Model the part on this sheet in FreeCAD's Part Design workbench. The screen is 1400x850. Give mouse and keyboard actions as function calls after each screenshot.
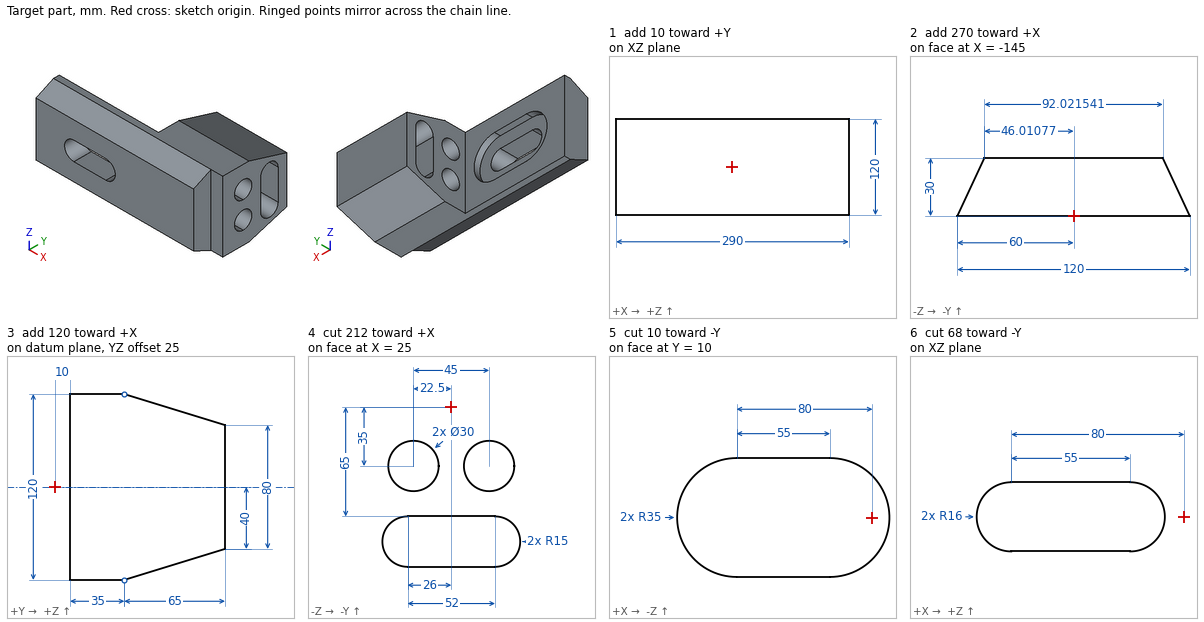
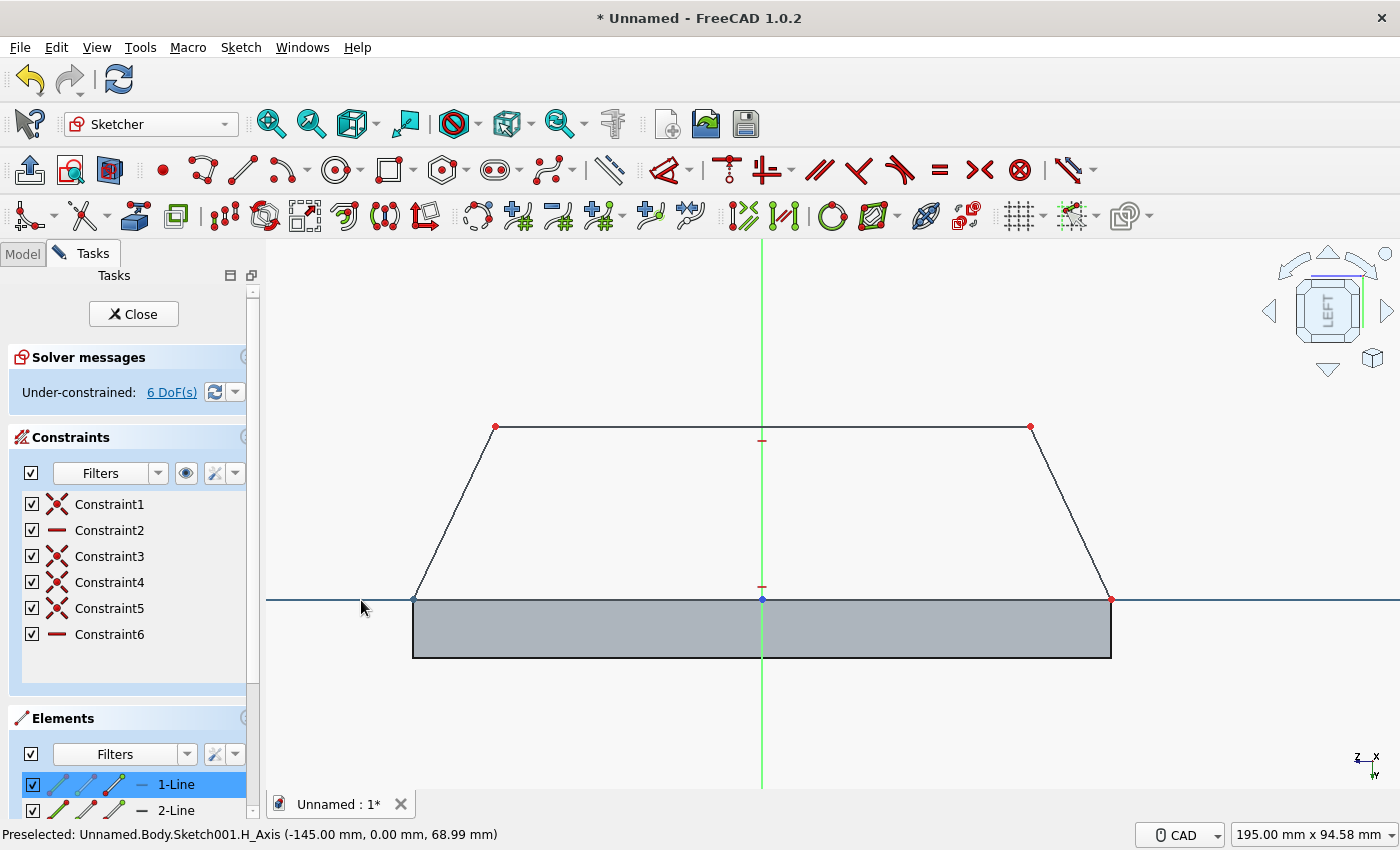
key(c)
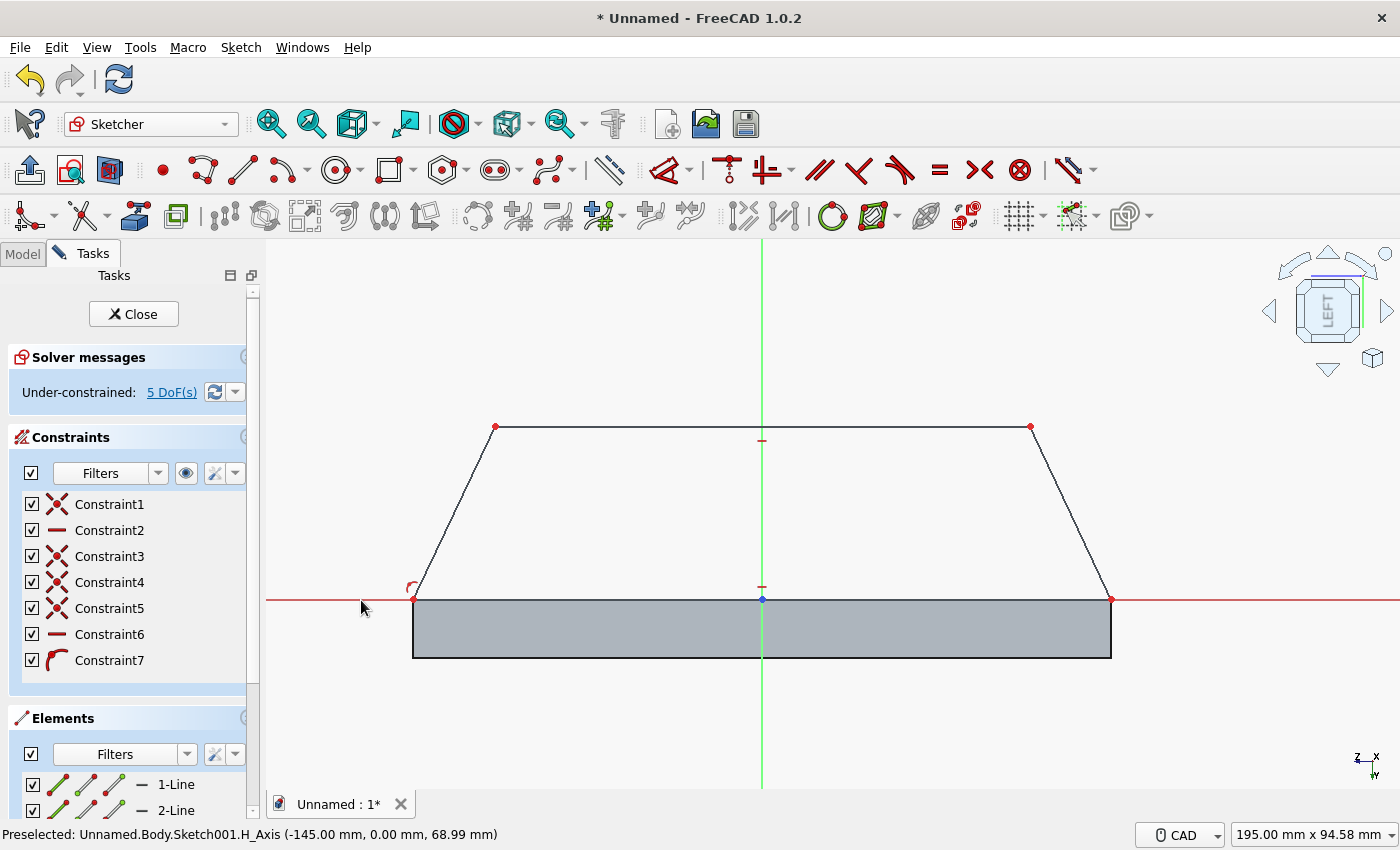
key(d)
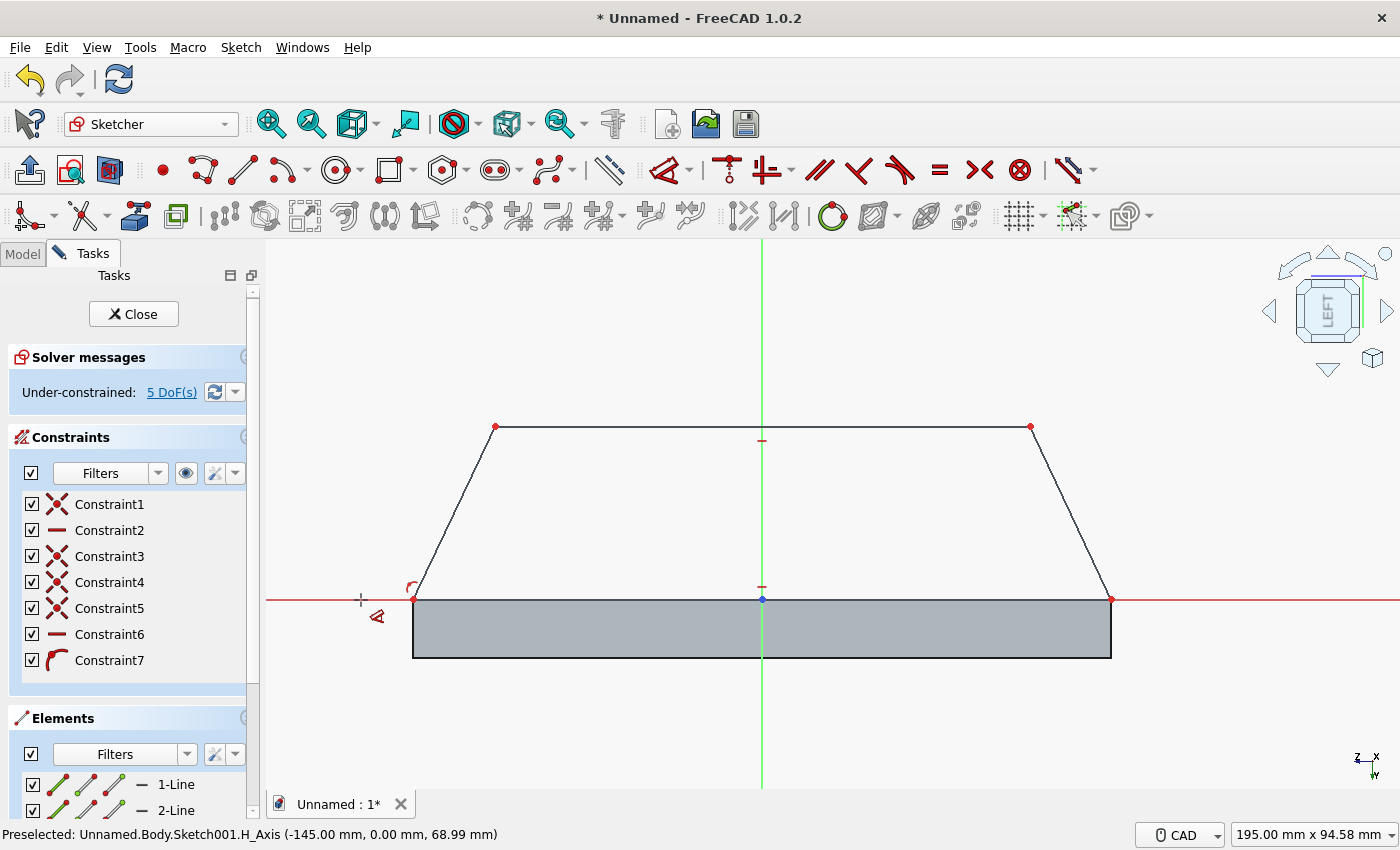
click(622, 600)
click(601, 634)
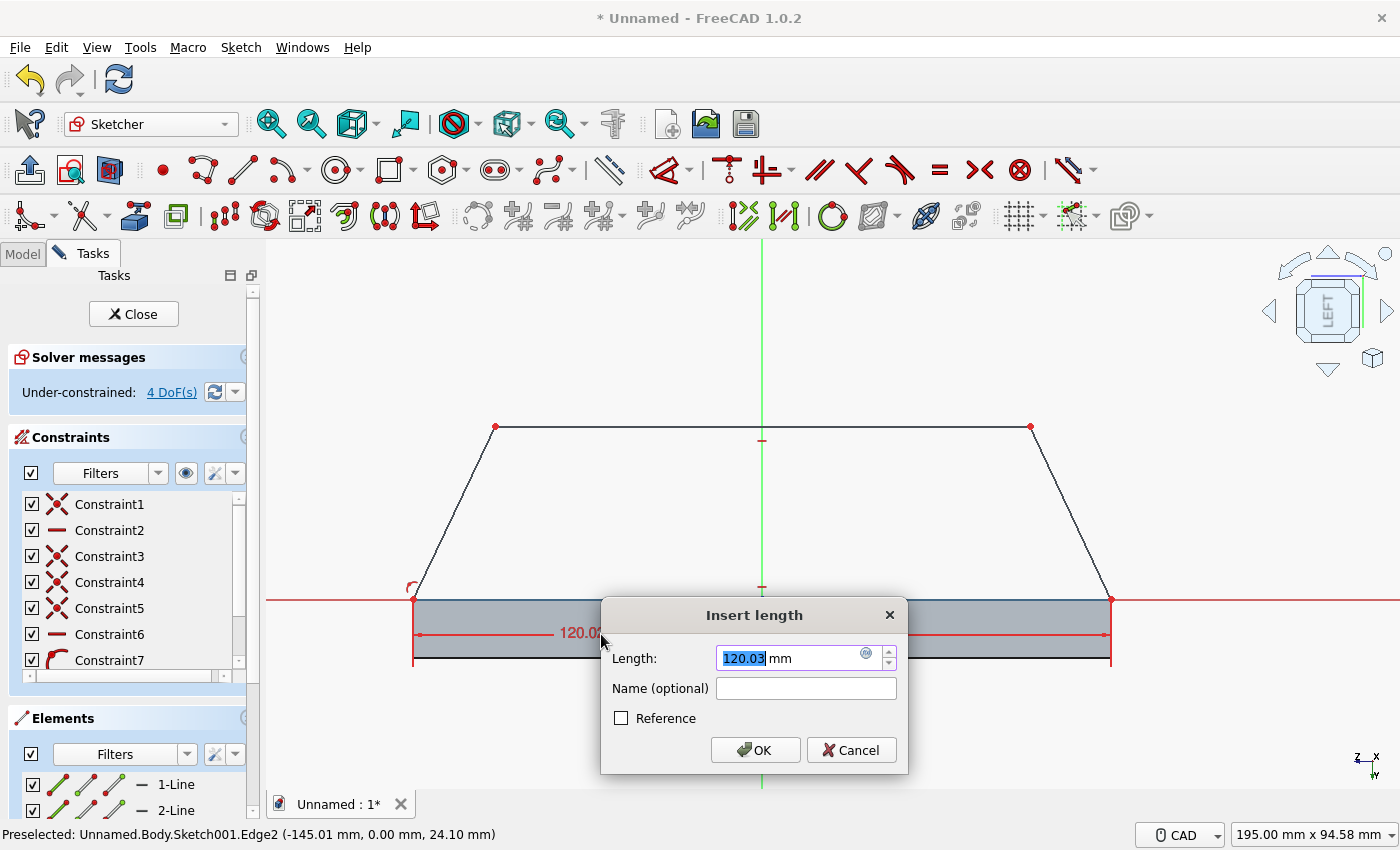
text(120)
key(Return)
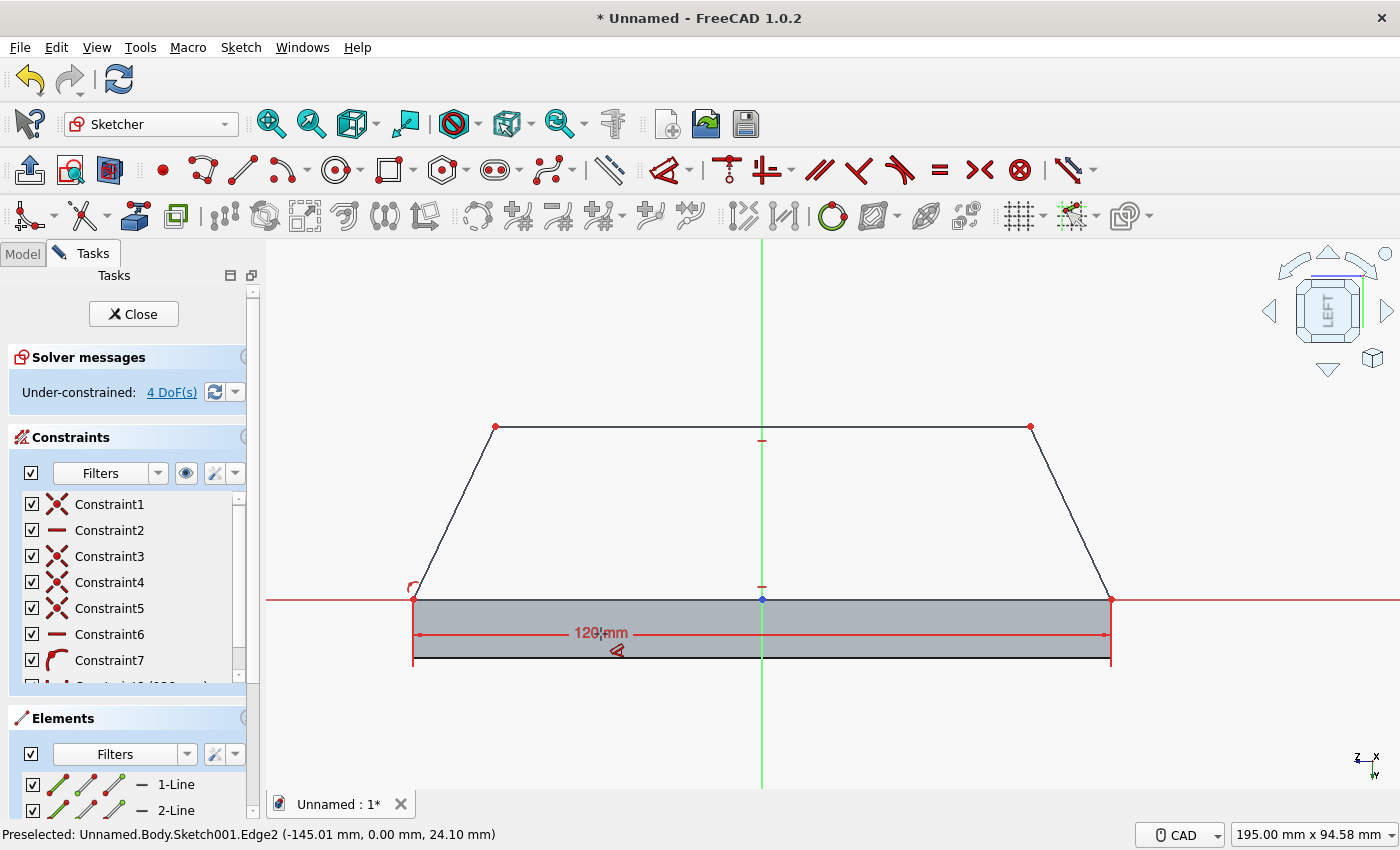
click(495, 427)
click(461, 553)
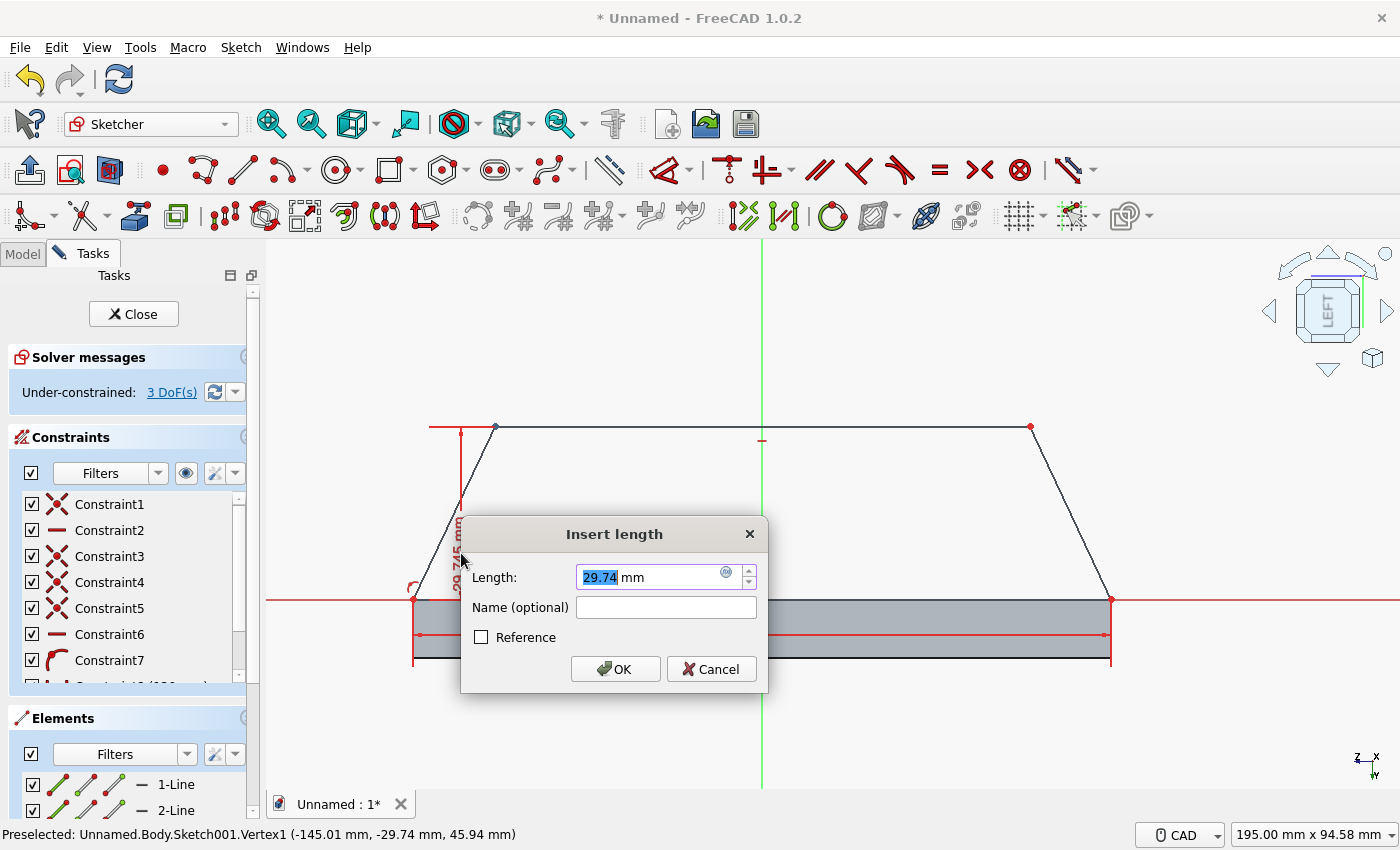
text(30)
key(Return)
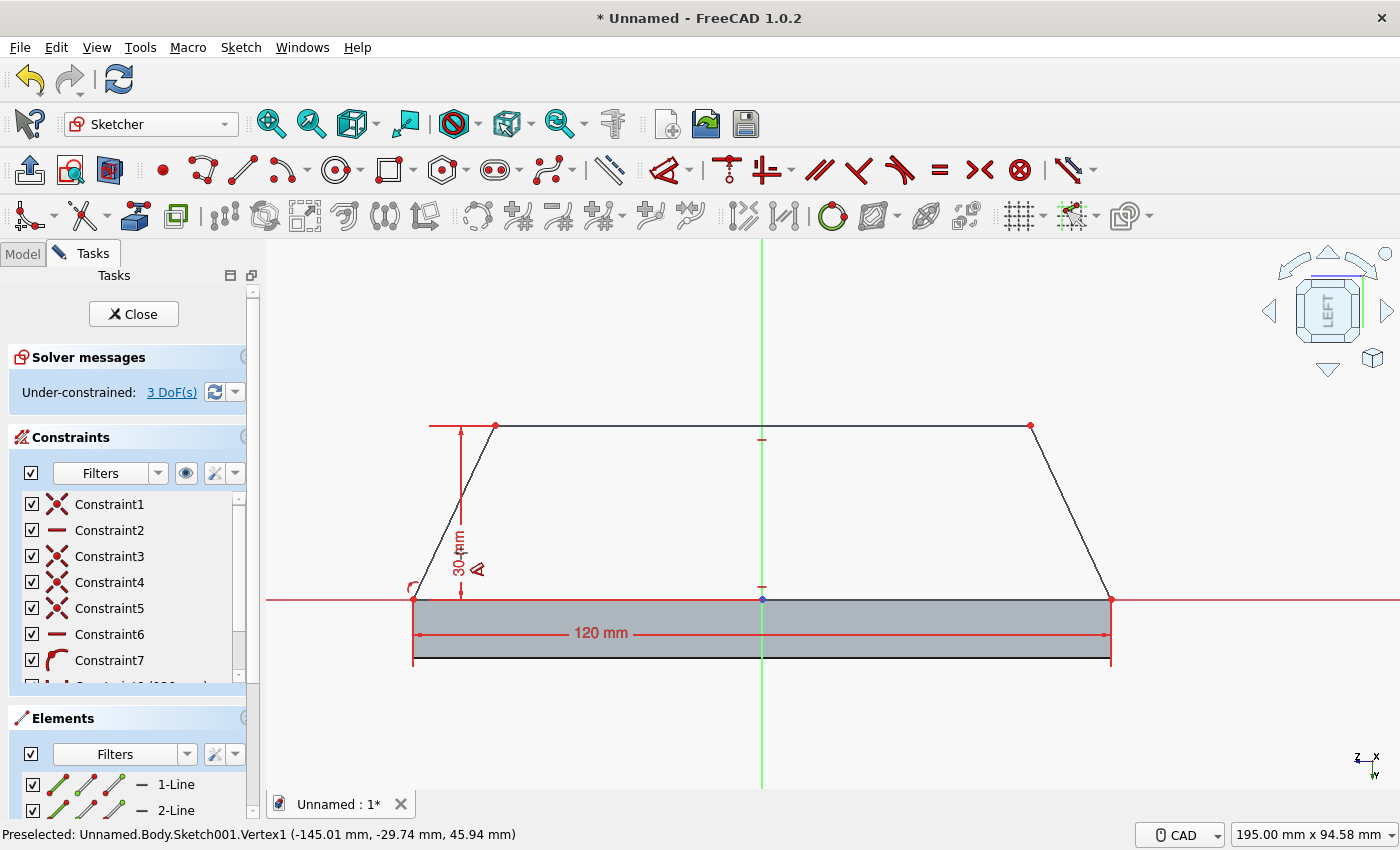
click(413, 600)
click(507, 634)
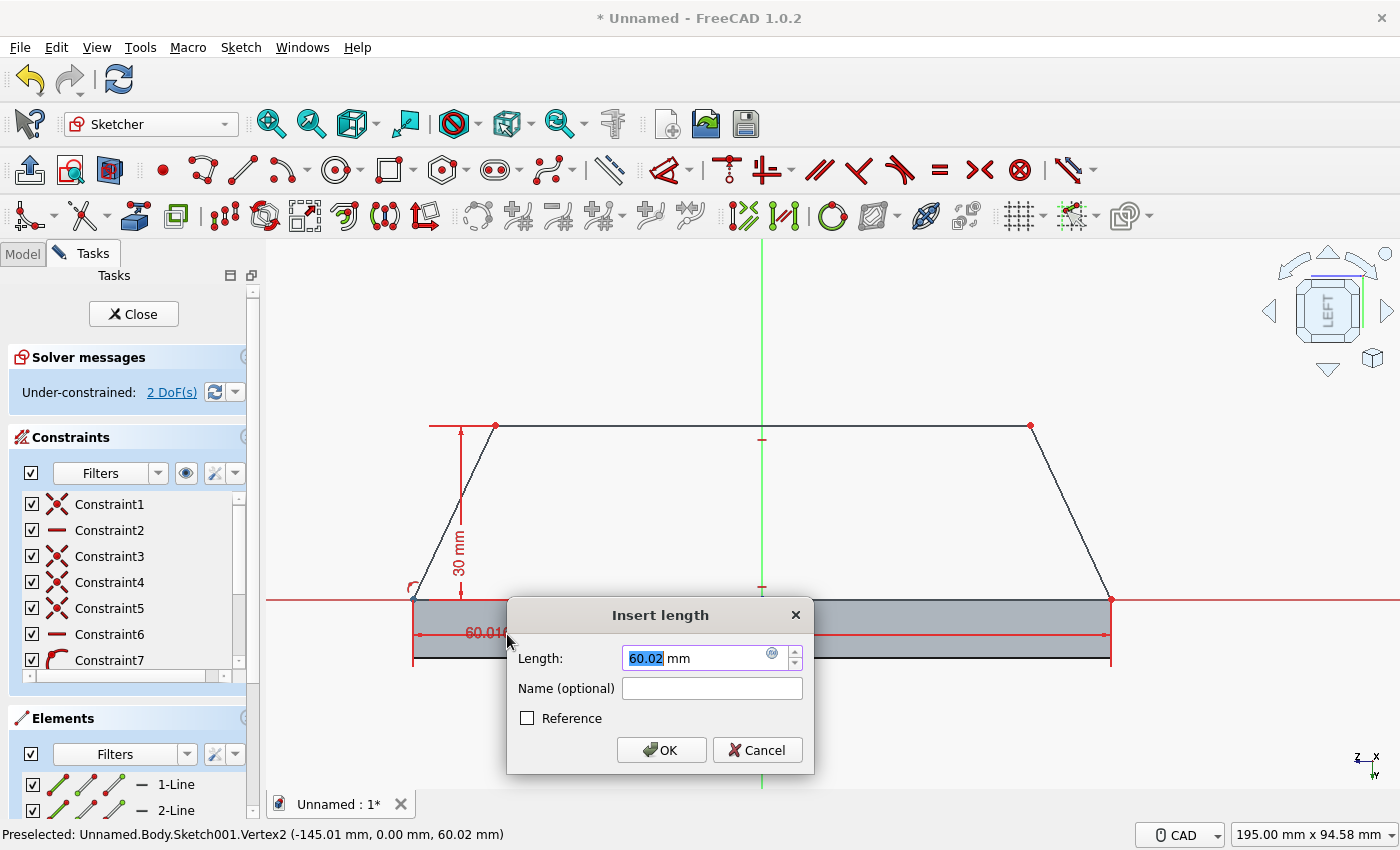
text(60)
key(Return)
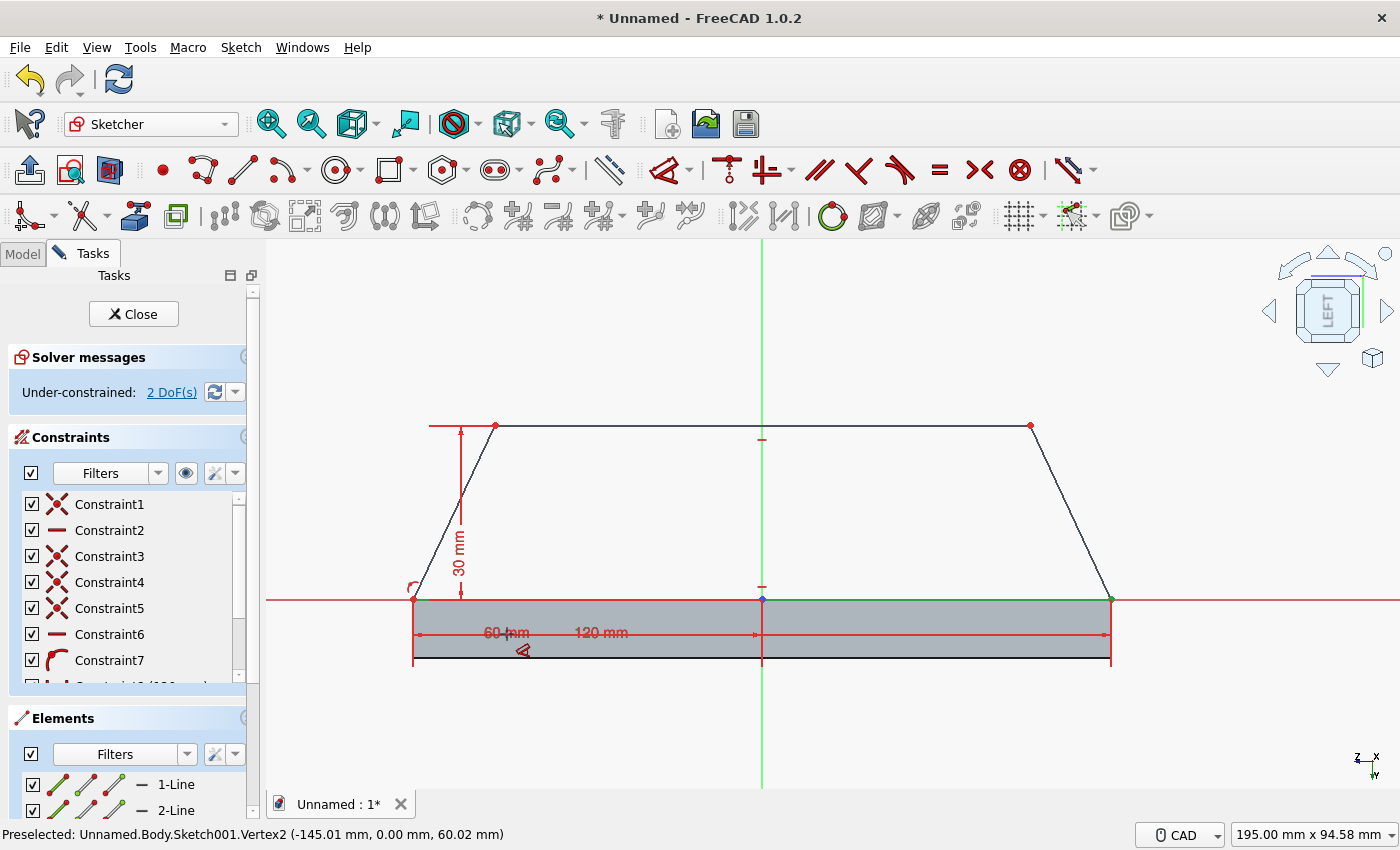
click(869, 426)
click(639, 392)